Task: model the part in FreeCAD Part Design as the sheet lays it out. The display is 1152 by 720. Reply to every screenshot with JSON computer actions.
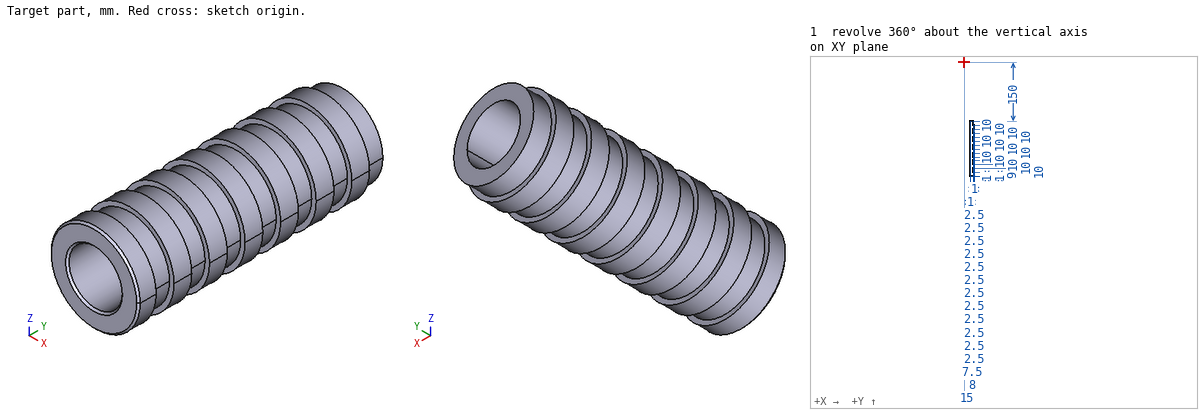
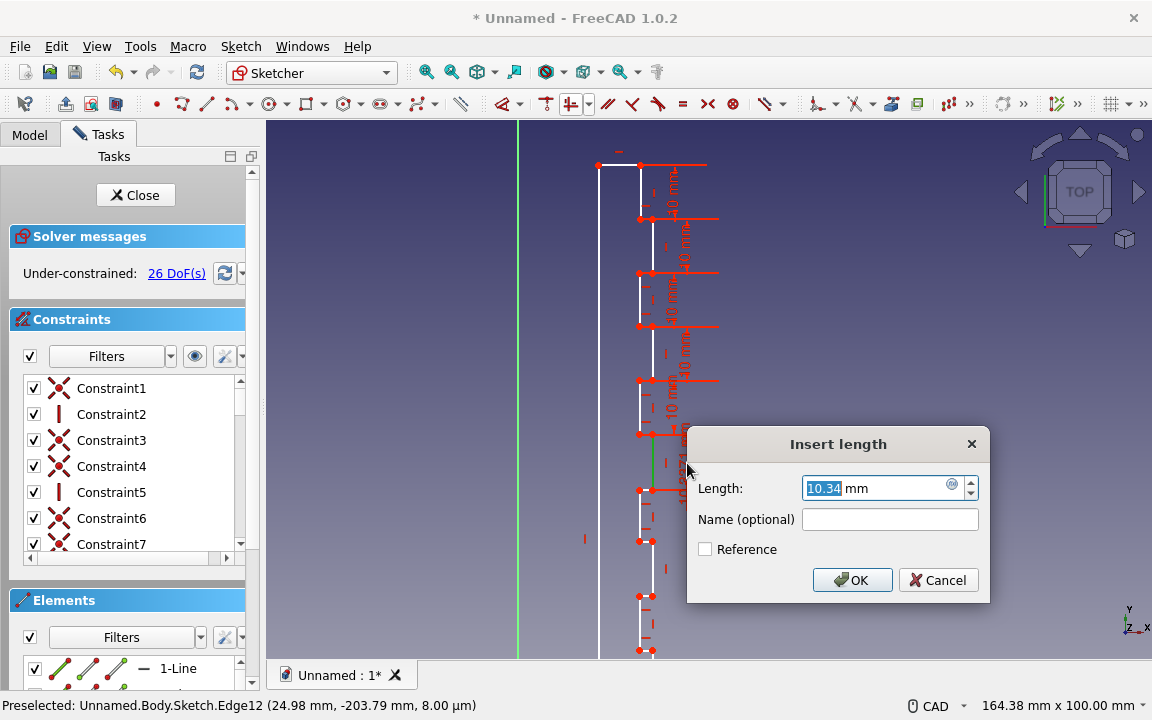
{"action": "type", "text": "10"}
{"action": "key", "text": "Return"}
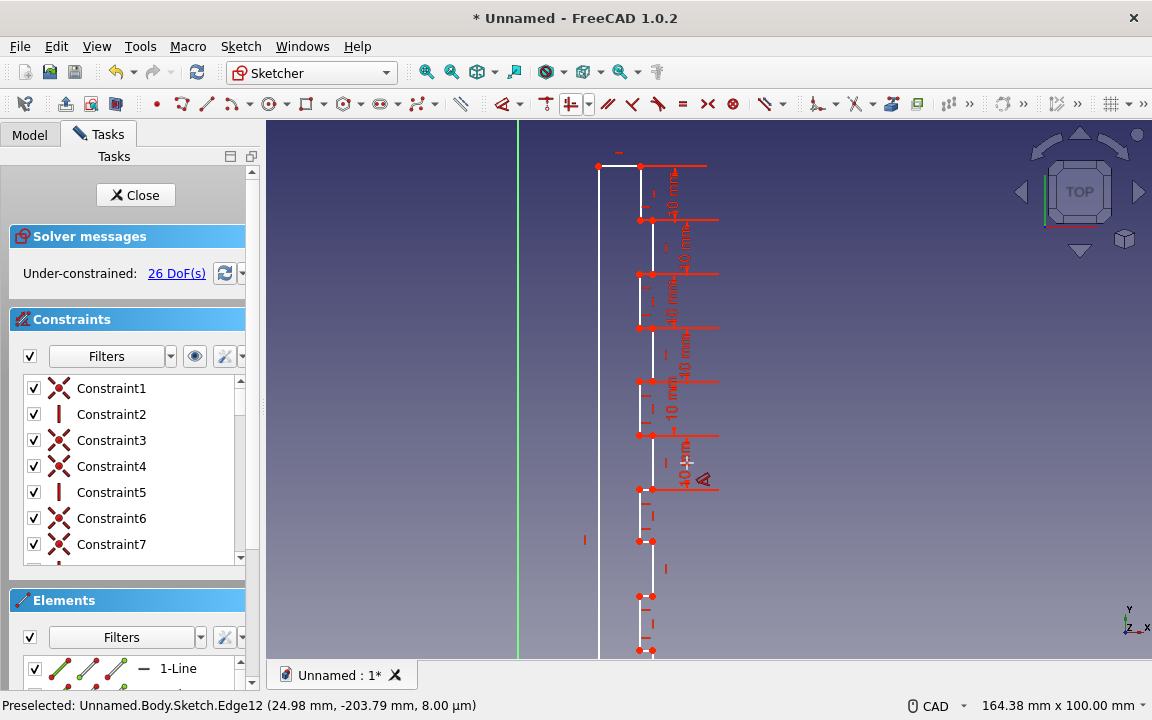
{"action": "left_click", "coordinate": [640, 505]}
{"action": "left_click", "coordinate": [674, 516]}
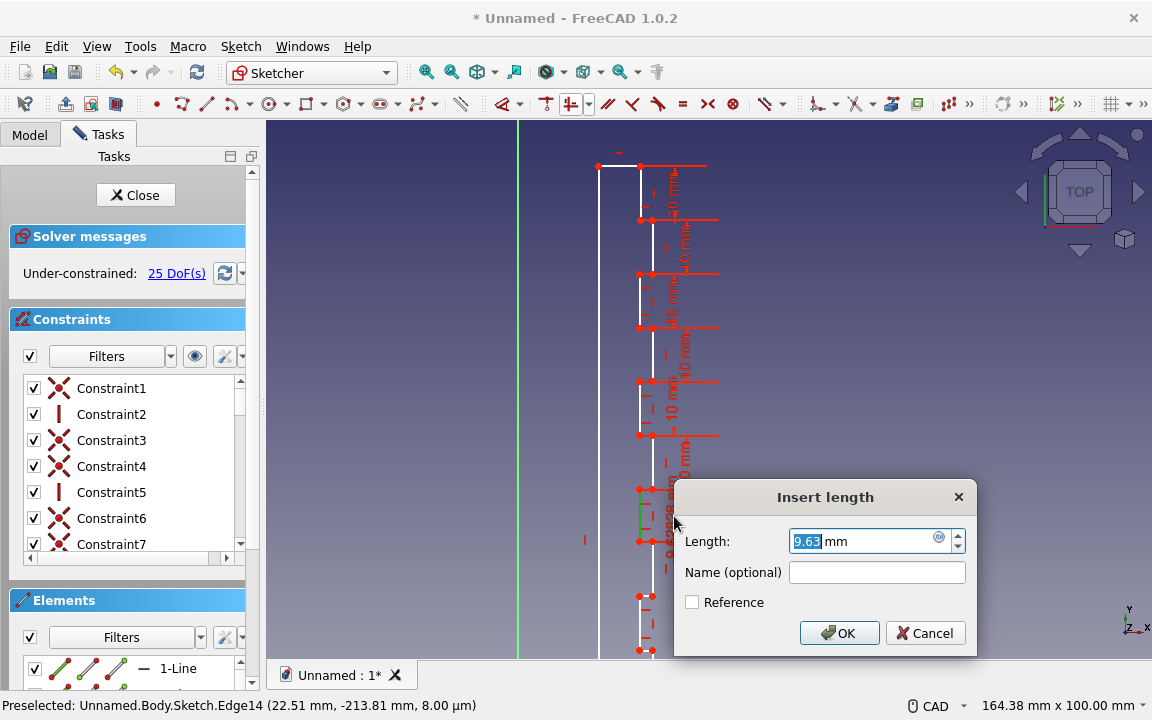
{"action": "type", "text": "10"}
{"action": "key", "text": "Return"}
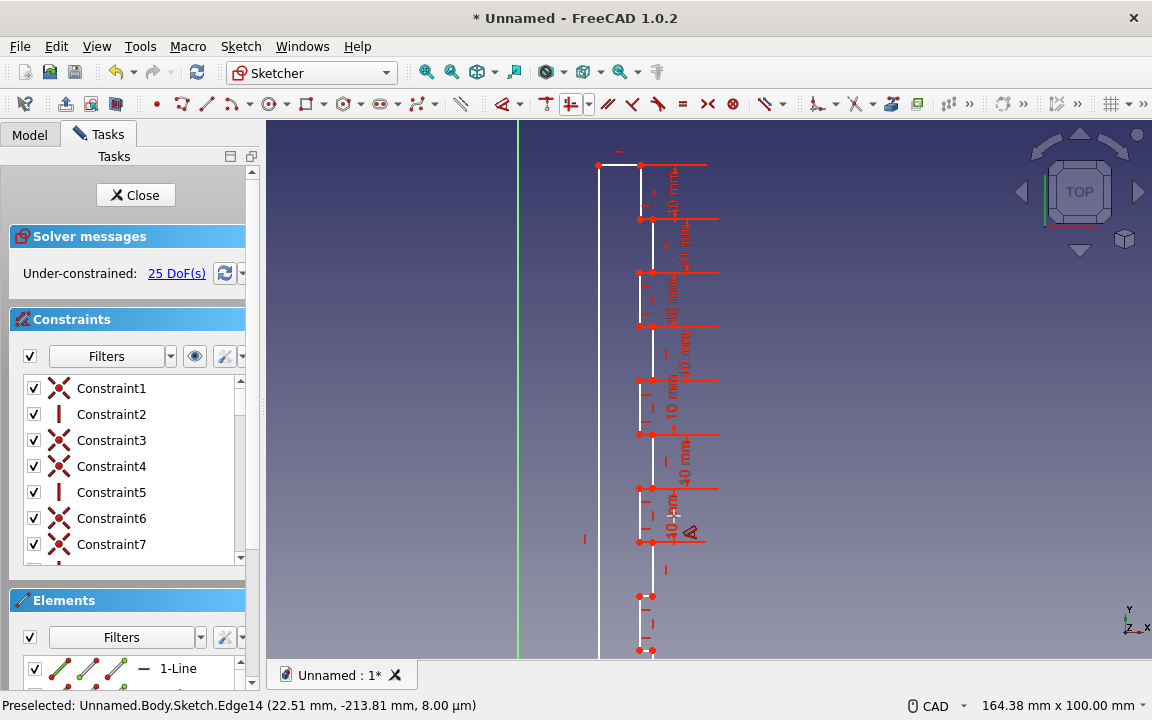
{"action": "left_click", "coordinate": [653, 559]}
{"action": "left_click", "coordinate": [687, 569]}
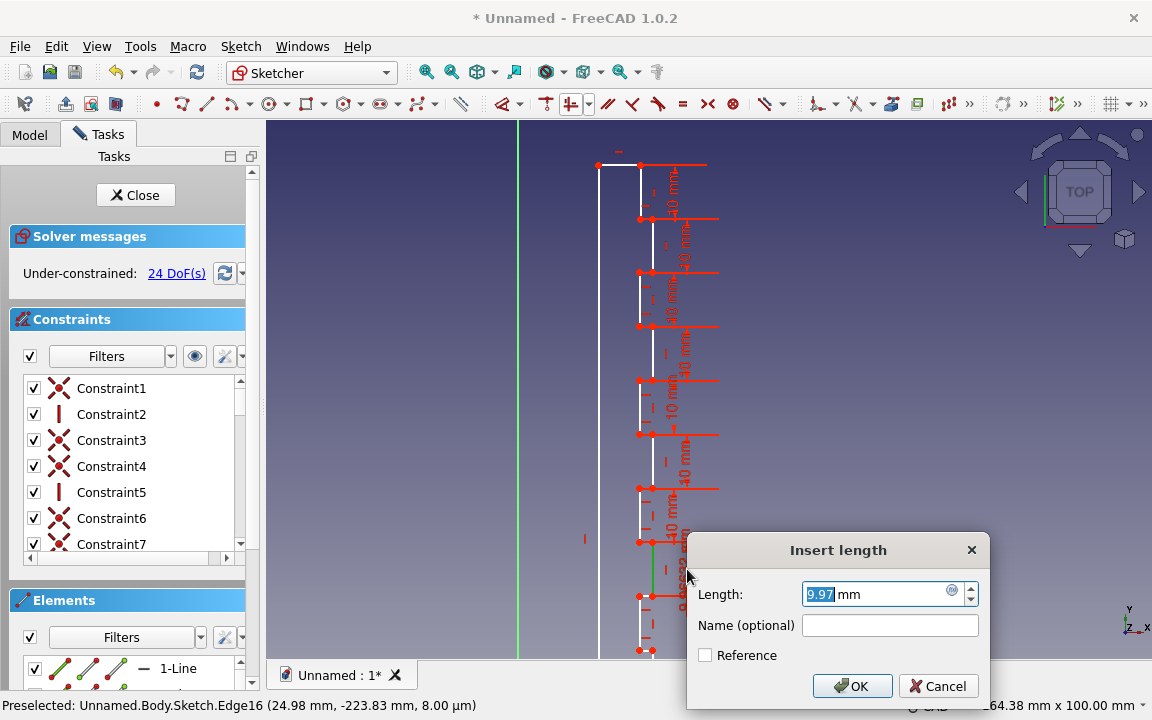
{"action": "type", "text": "10"}
{"action": "key", "text": "Return"}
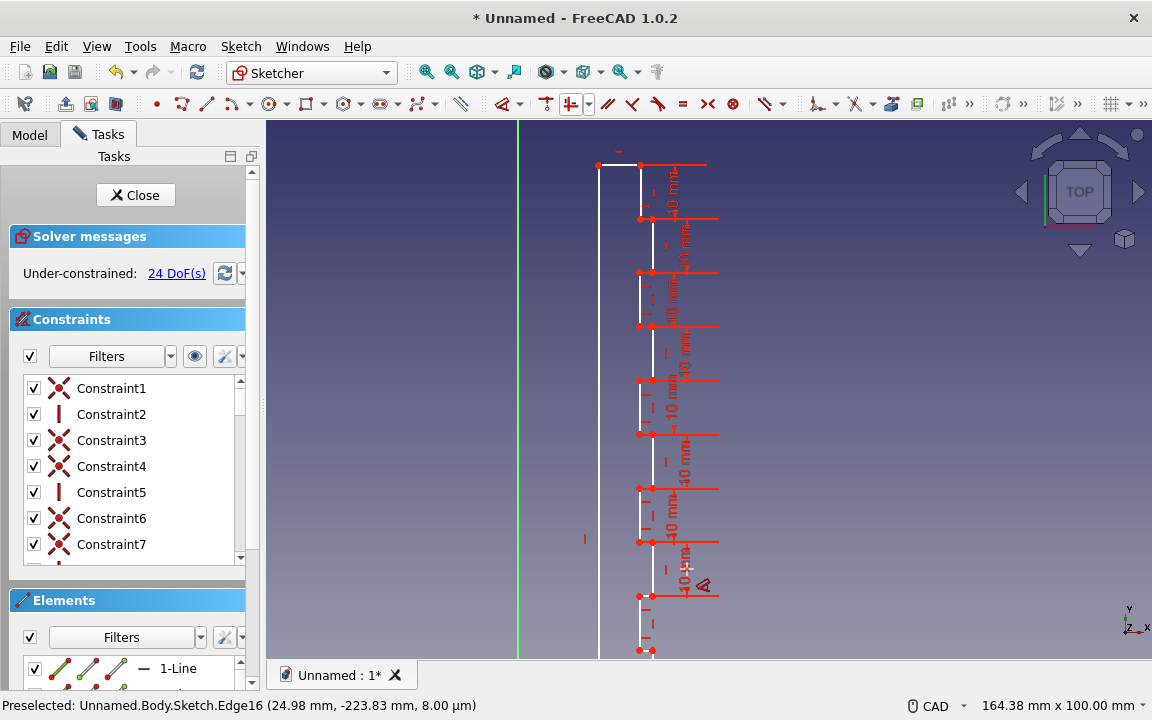
{"action": "left_click", "coordinate": [640, 613]}
{"action": "left_click", "coordinate": [674, 614]}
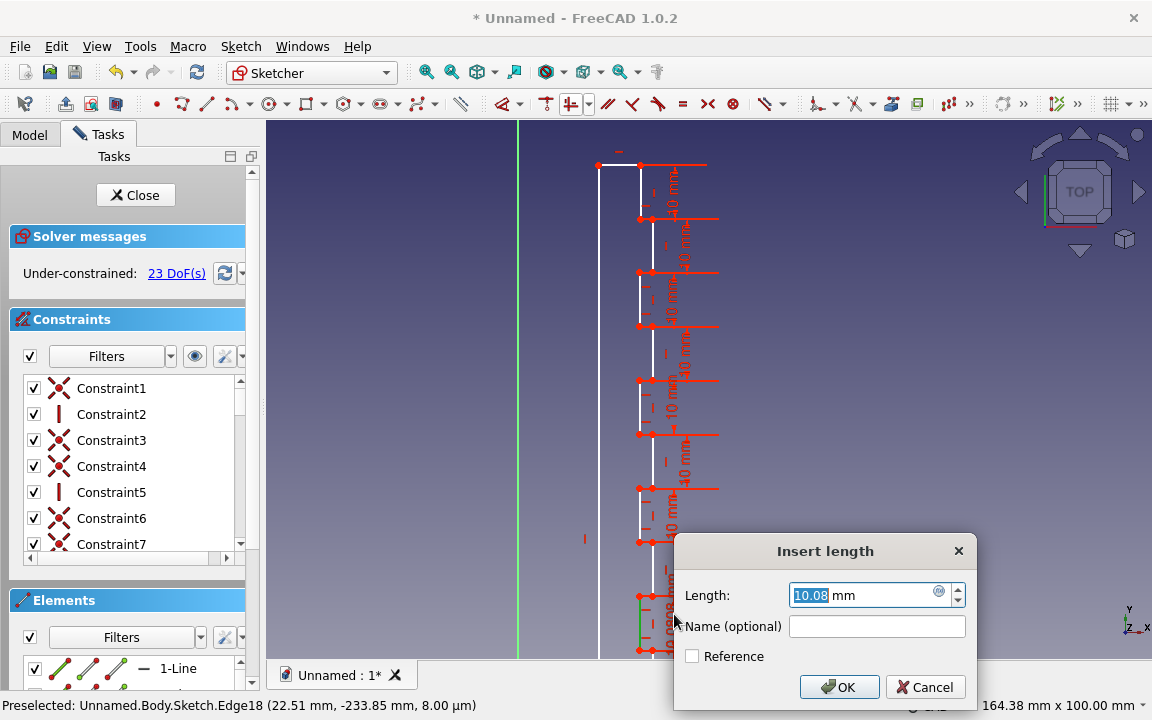
{"action": "type", "text": "10"}
{"action": "key", "text": "Return"}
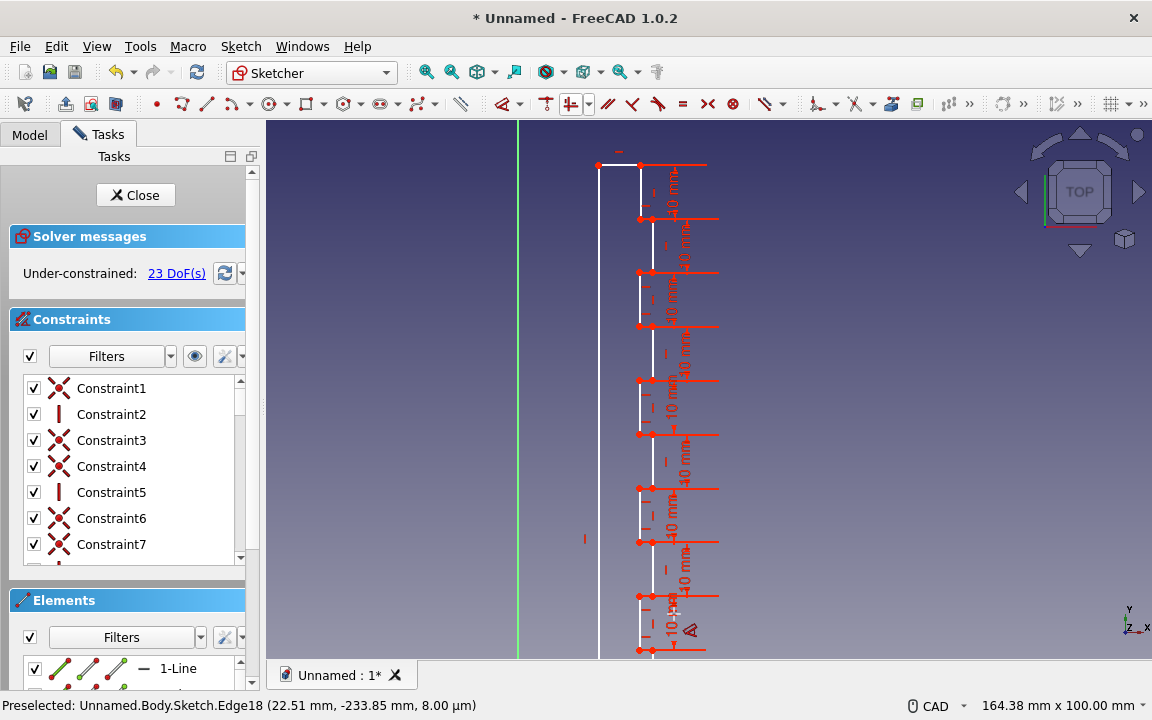
{"action": "scroll", "coordinate": [654, 454], "scroll_direction": "down", "scroll_amount": 8}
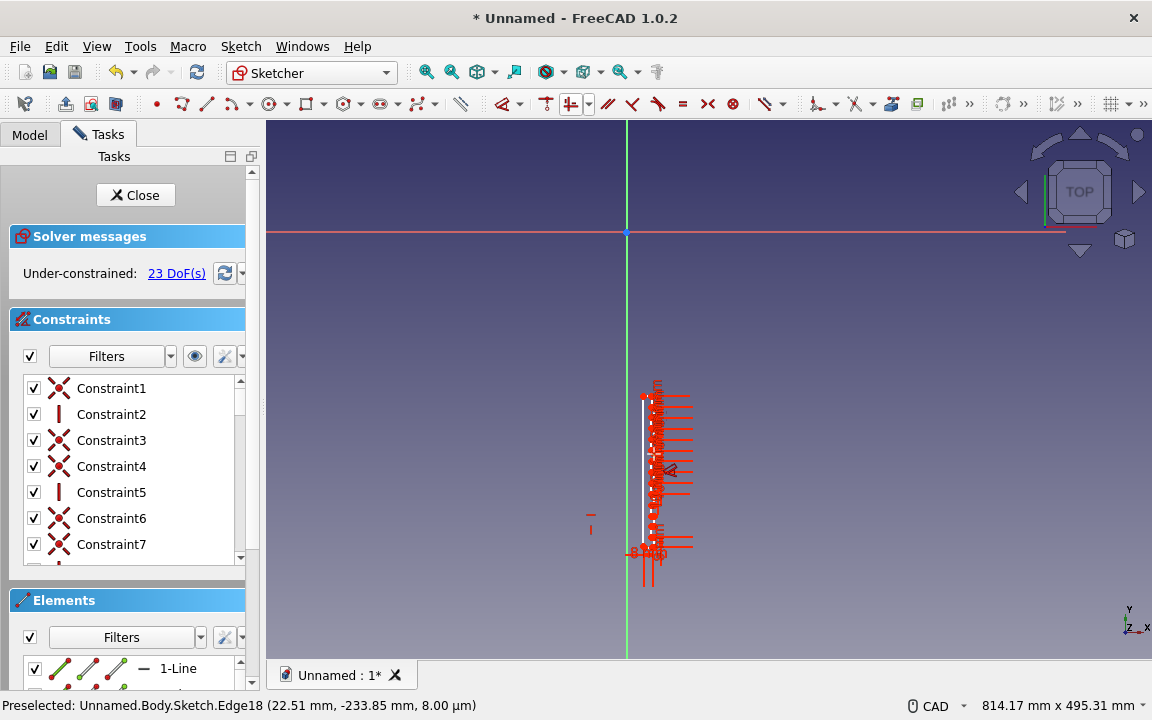
{"action": "scroll", "coordinate": [654, 497], "scroll_direction": "up", "scroll_amount": 8}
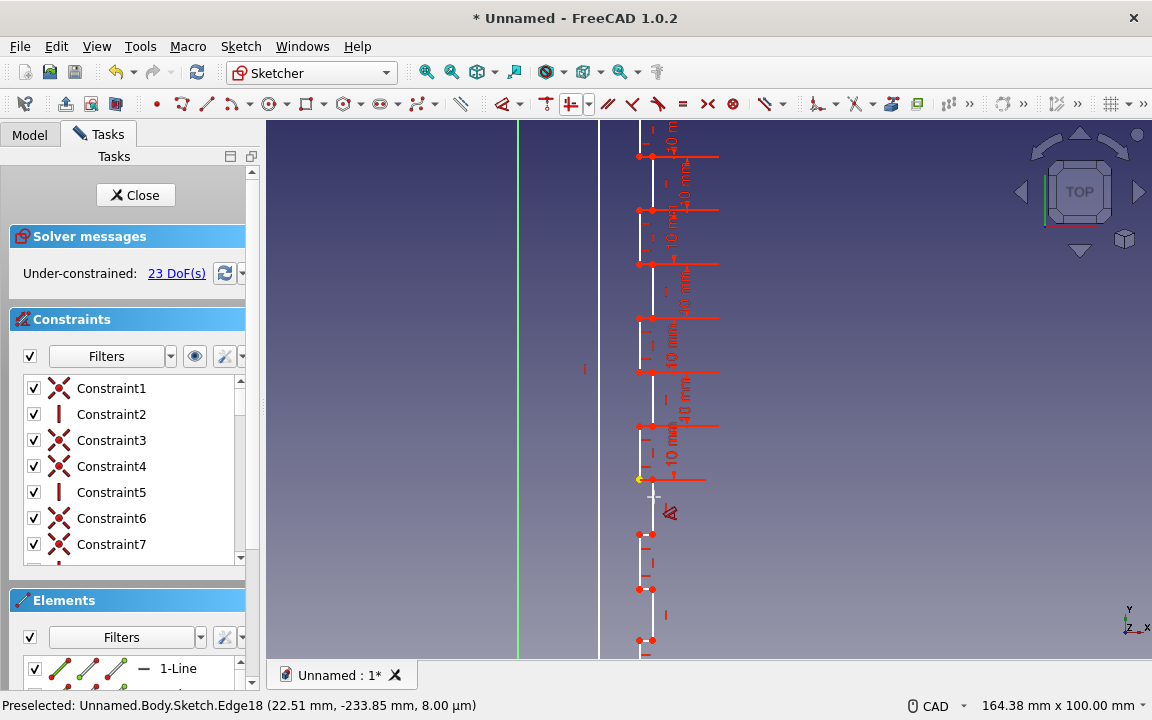
{"action": "left_click", "coordinate": [653, 496]}
{"action": "left_click", "coordinate": [687, 507]}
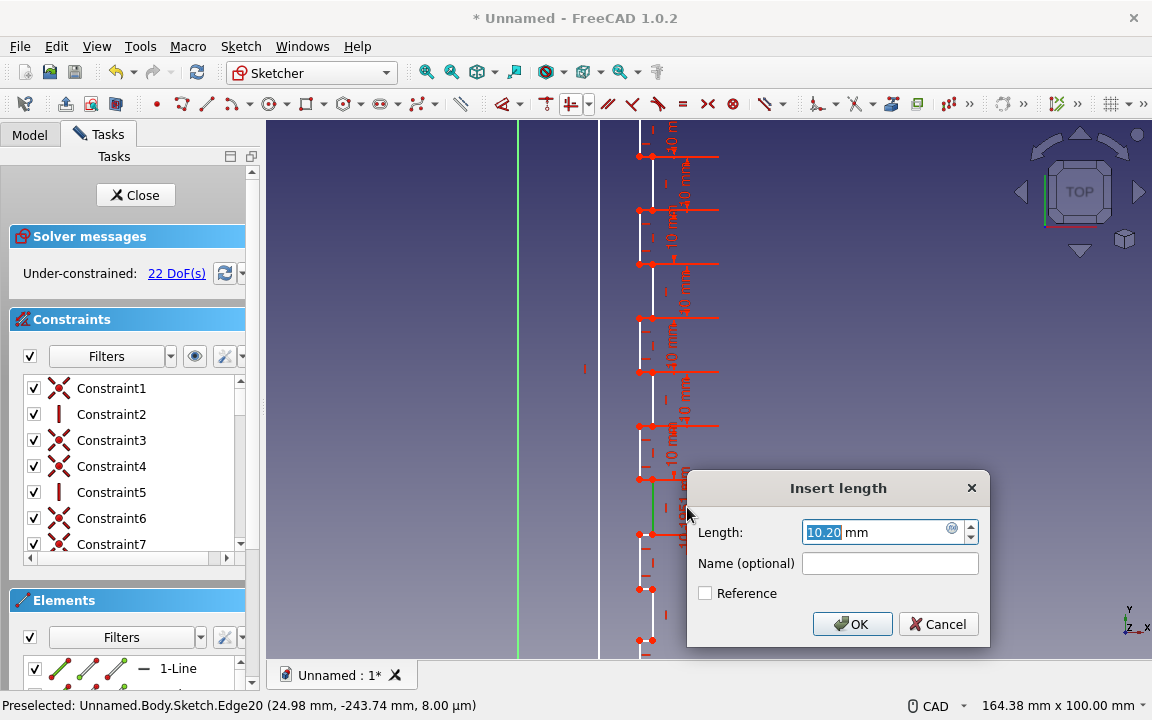
{"action": "type", "text": "10"}
{"action": "key", "text": "Return"}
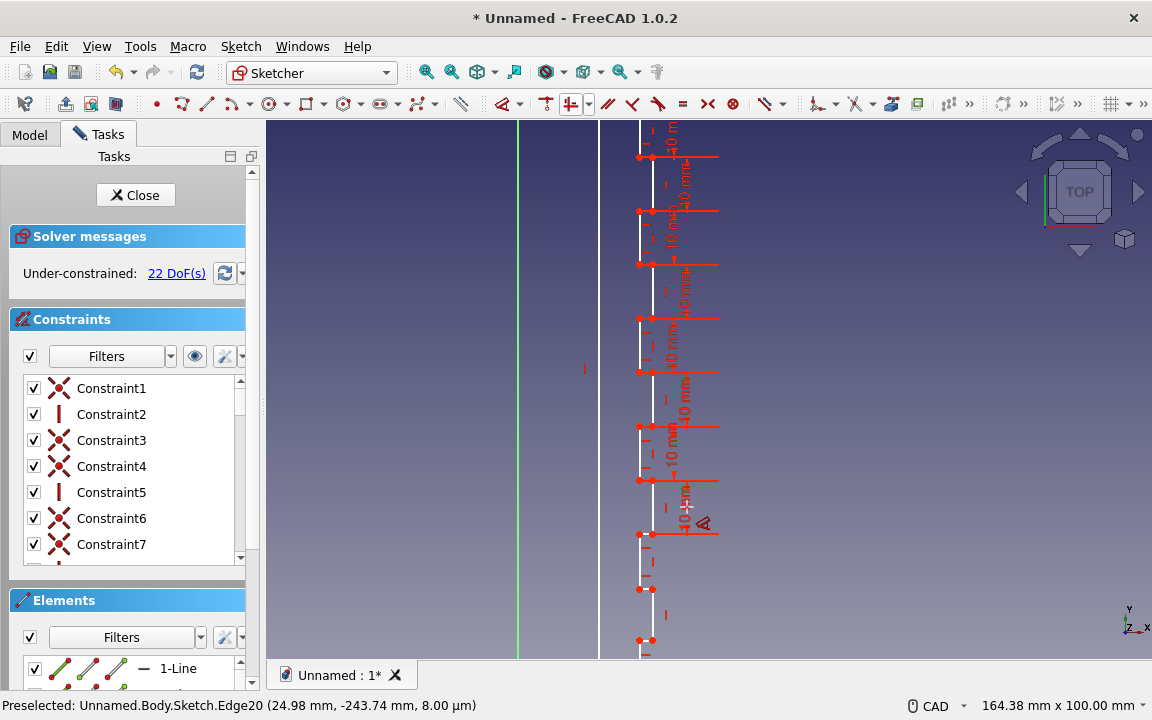
{"action": "left_click", "coordinate": [640, 551]}
{"action": "left_click", "coordinate": [674, 562]}